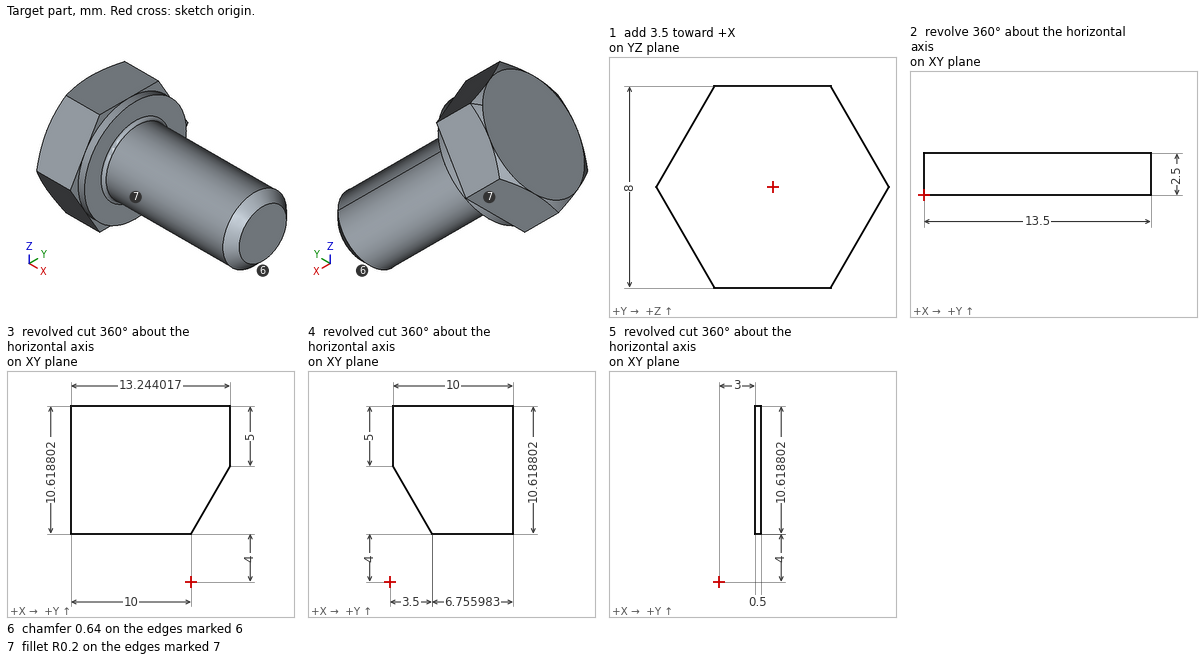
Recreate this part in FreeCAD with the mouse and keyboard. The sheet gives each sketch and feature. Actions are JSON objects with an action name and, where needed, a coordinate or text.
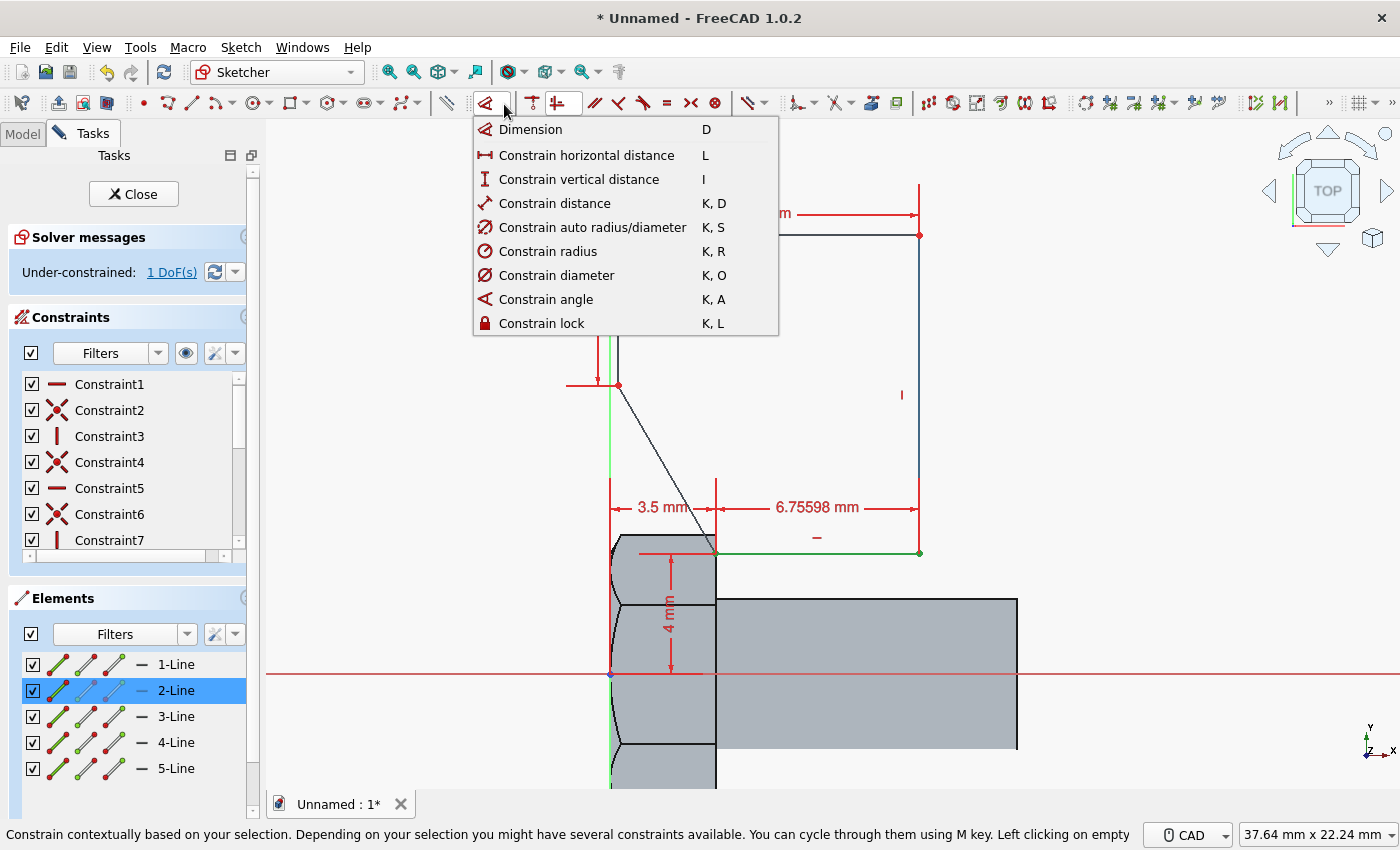
{"action": "left_click", "coordinate": [626, 179]}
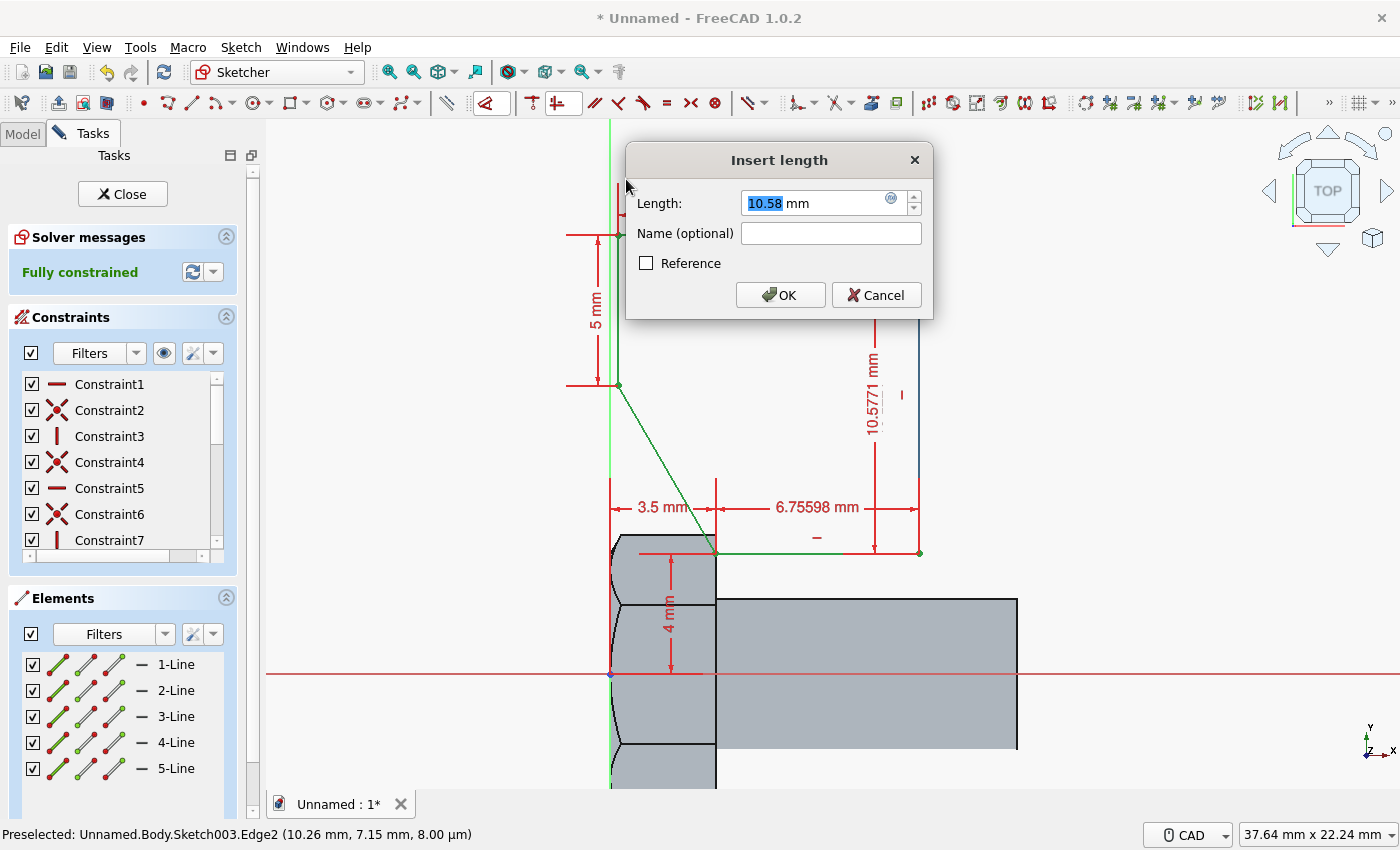
{"action": "type", "text": "10.618802"}
{"action": "key", "text": "Return"}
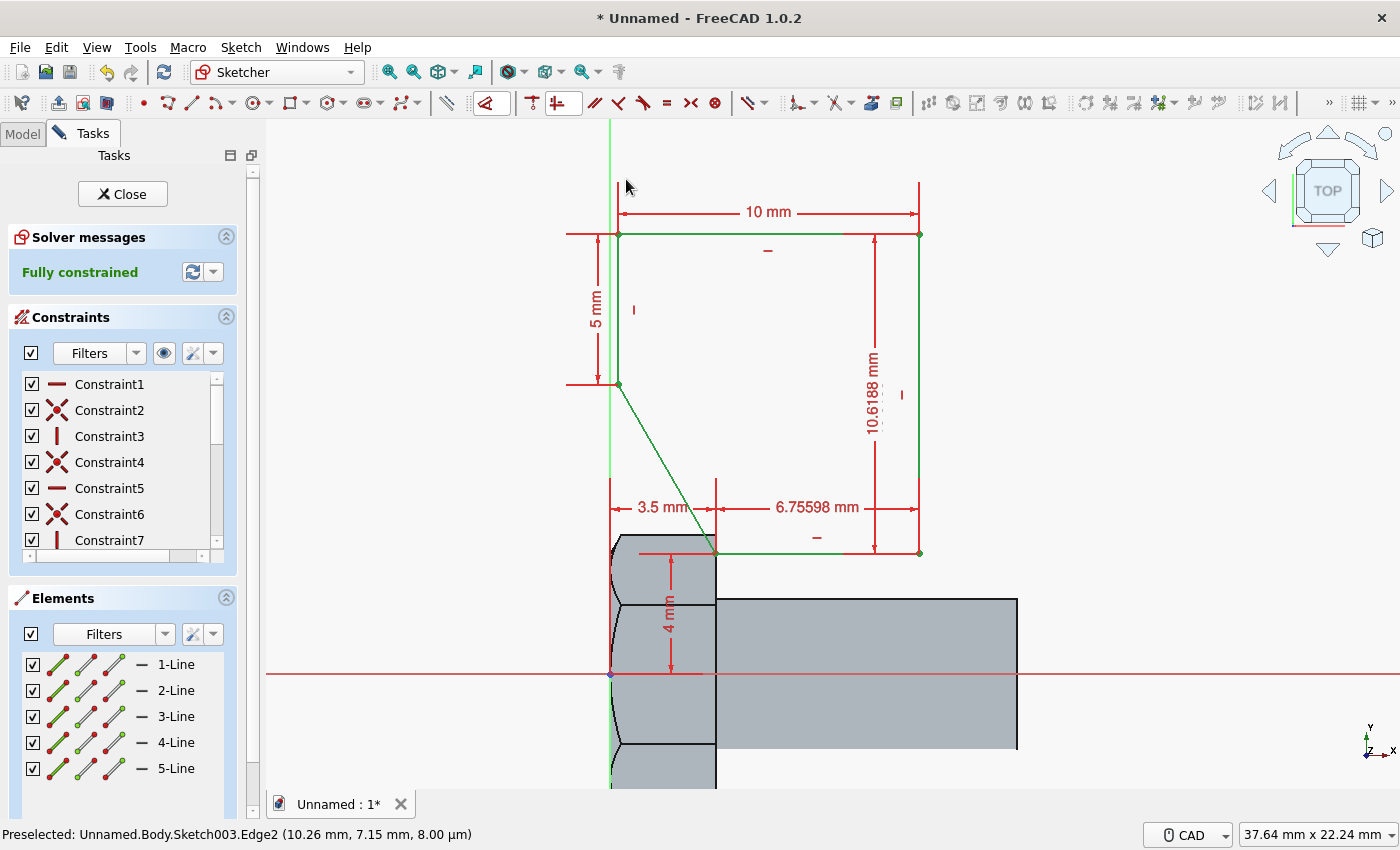
{"action": "left_click", "coordinate": [123, 194]}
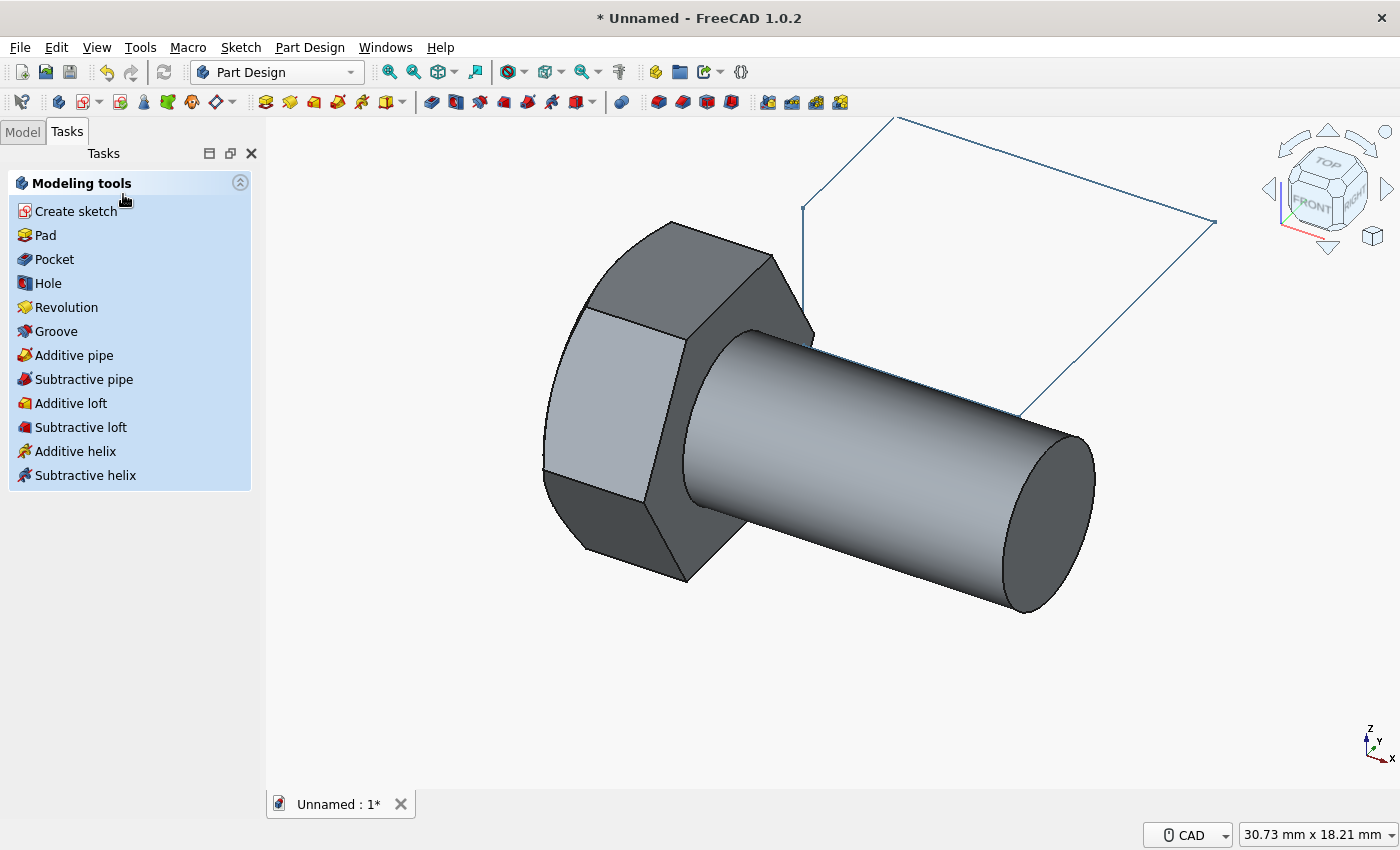
{"action": "left_click", "coordinate": [480, 102]}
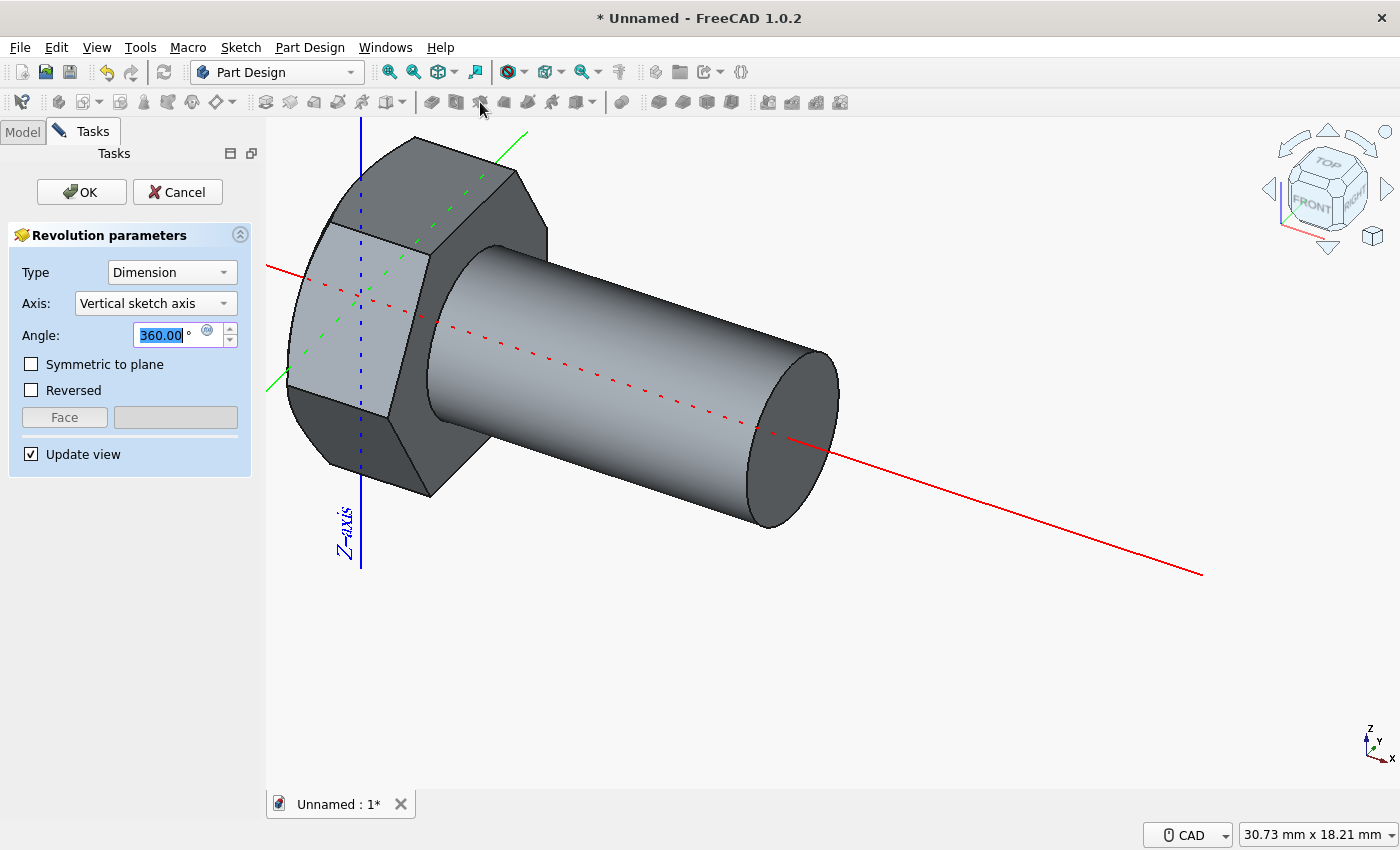
{"action": "left_click", "coordinate": [156, 304]}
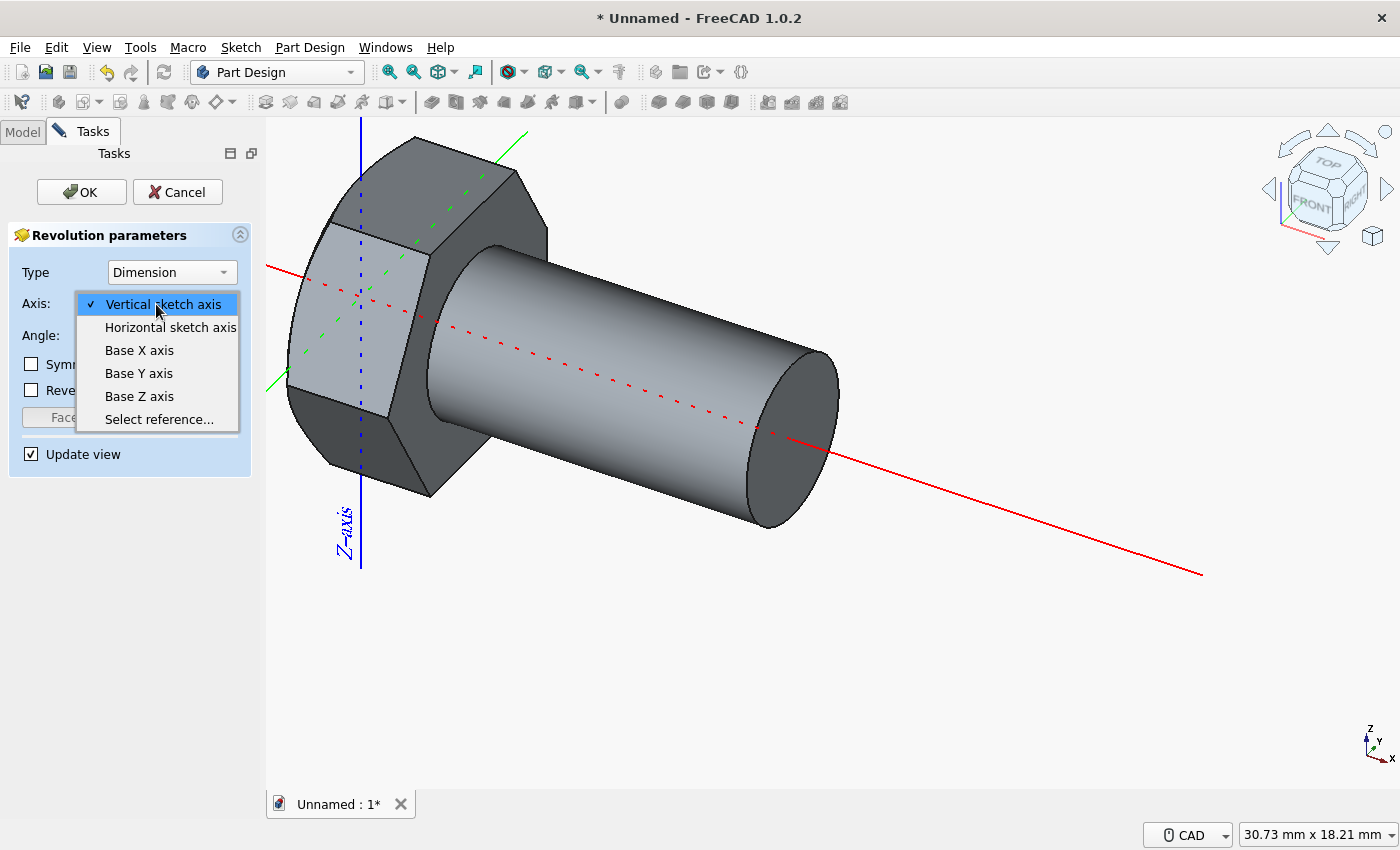
{"action": "left_click", "coordinate": [156, 328]}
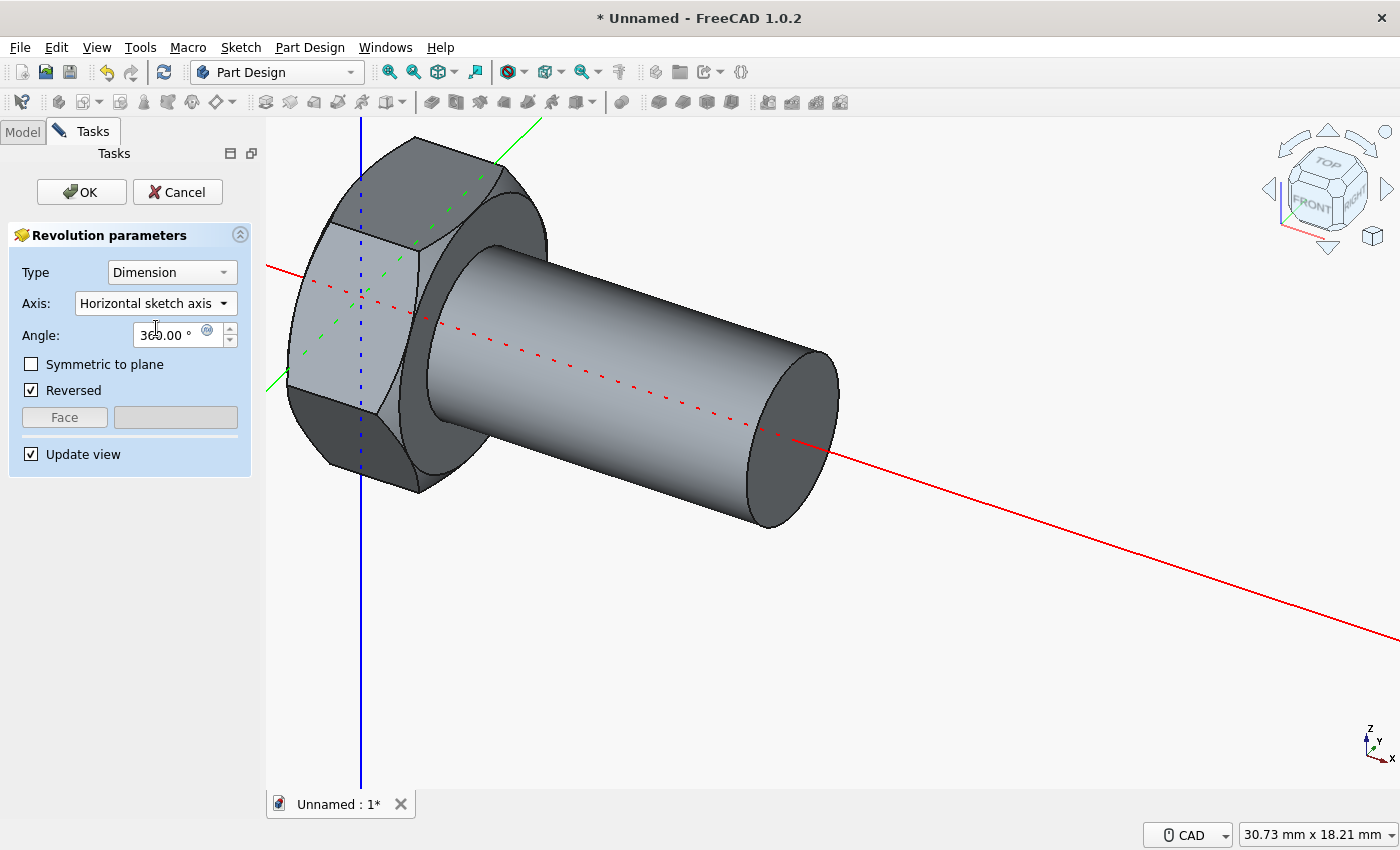
{"action": "left_click", "coordinate": [82, 192]}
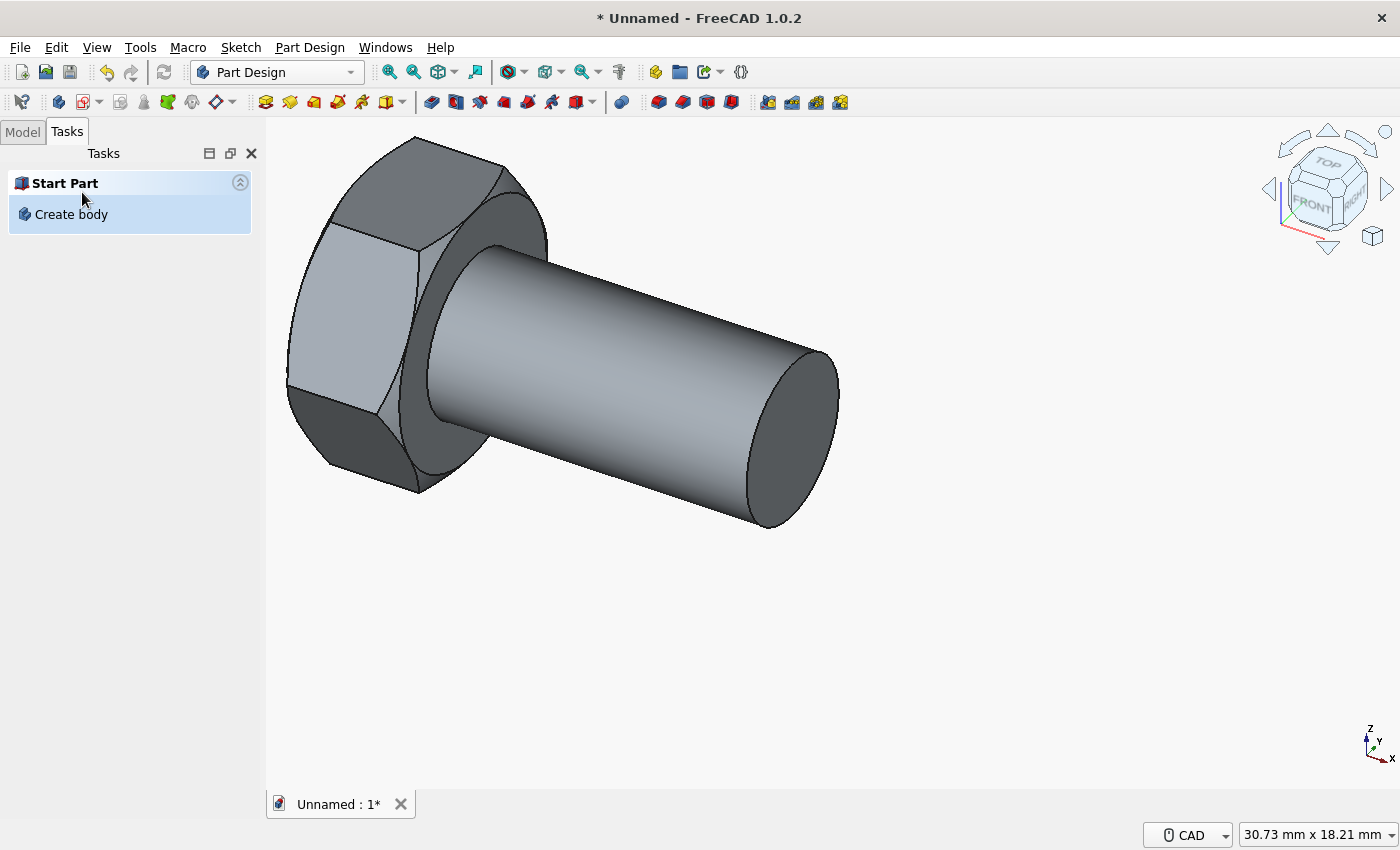
{"action": "left_click", "coordinate": [390, 72]}